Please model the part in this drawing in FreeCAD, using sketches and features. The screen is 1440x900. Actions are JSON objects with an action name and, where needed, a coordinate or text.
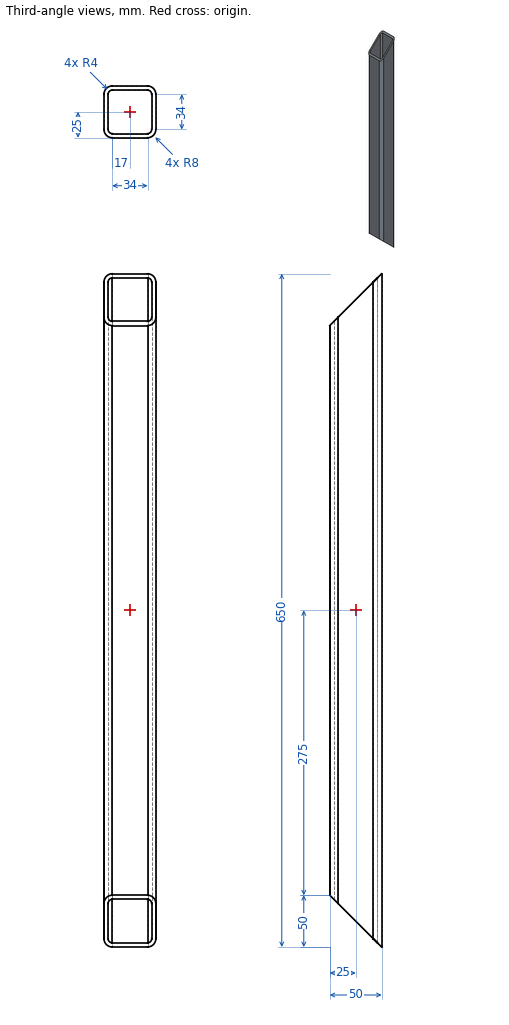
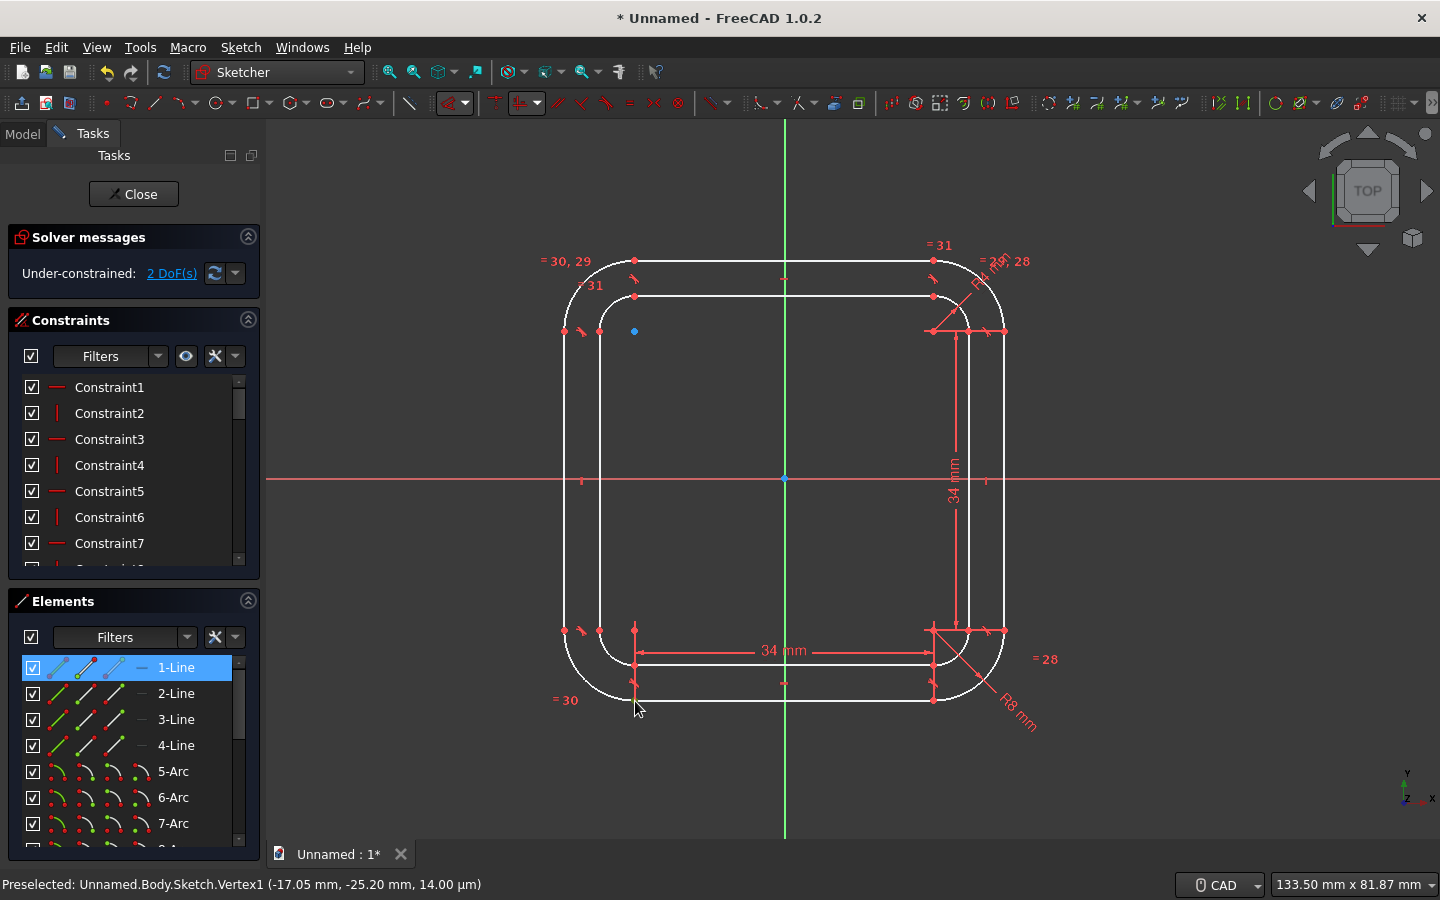
{"action": "key", "text": "l"}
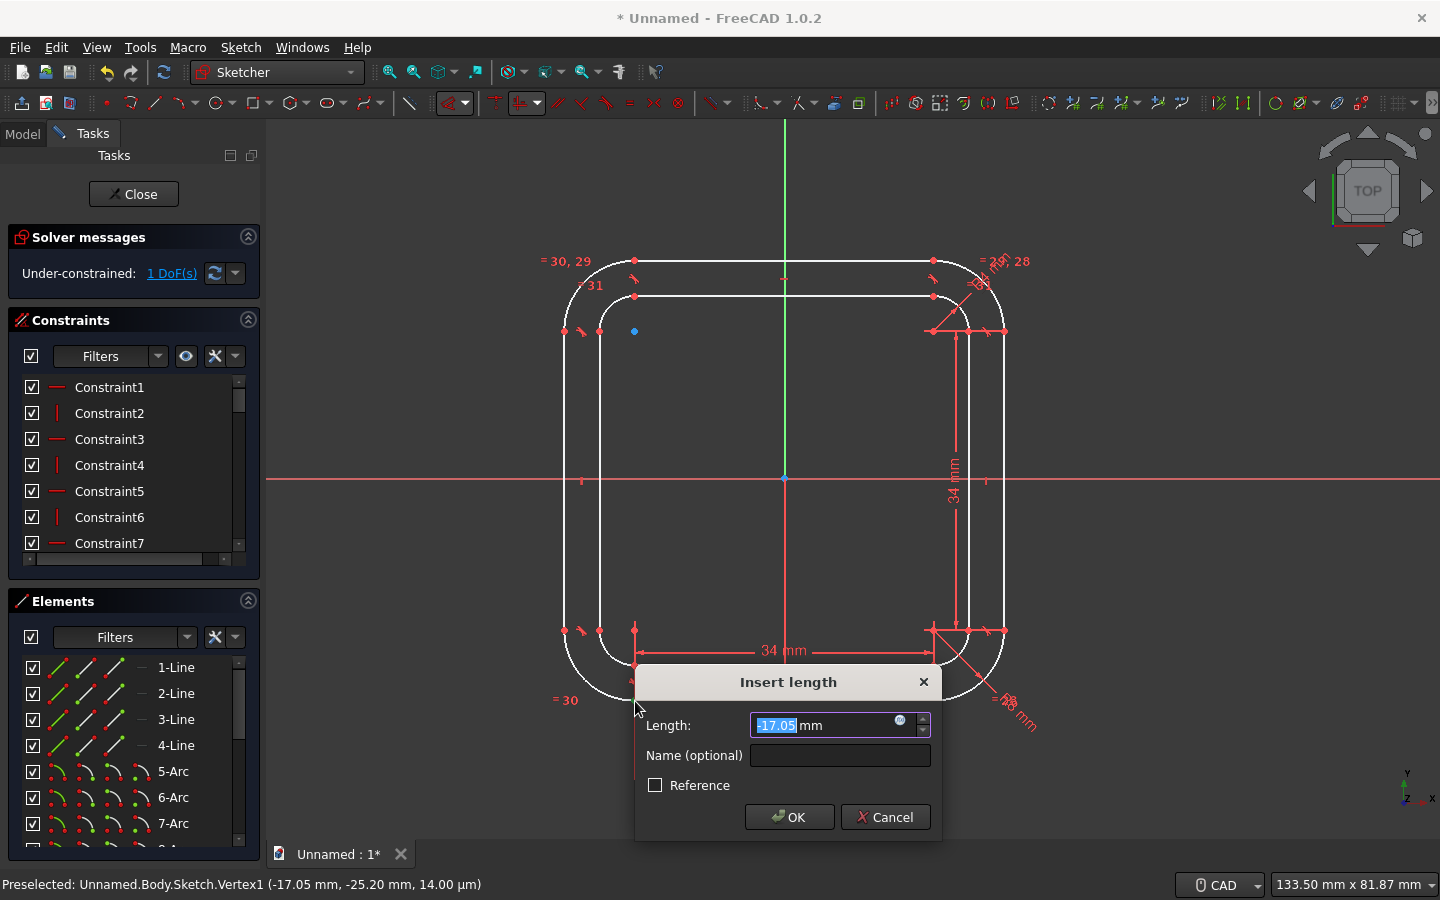
{"action": "type", "text": "-17"}
{"action": "key", "text": "Return"}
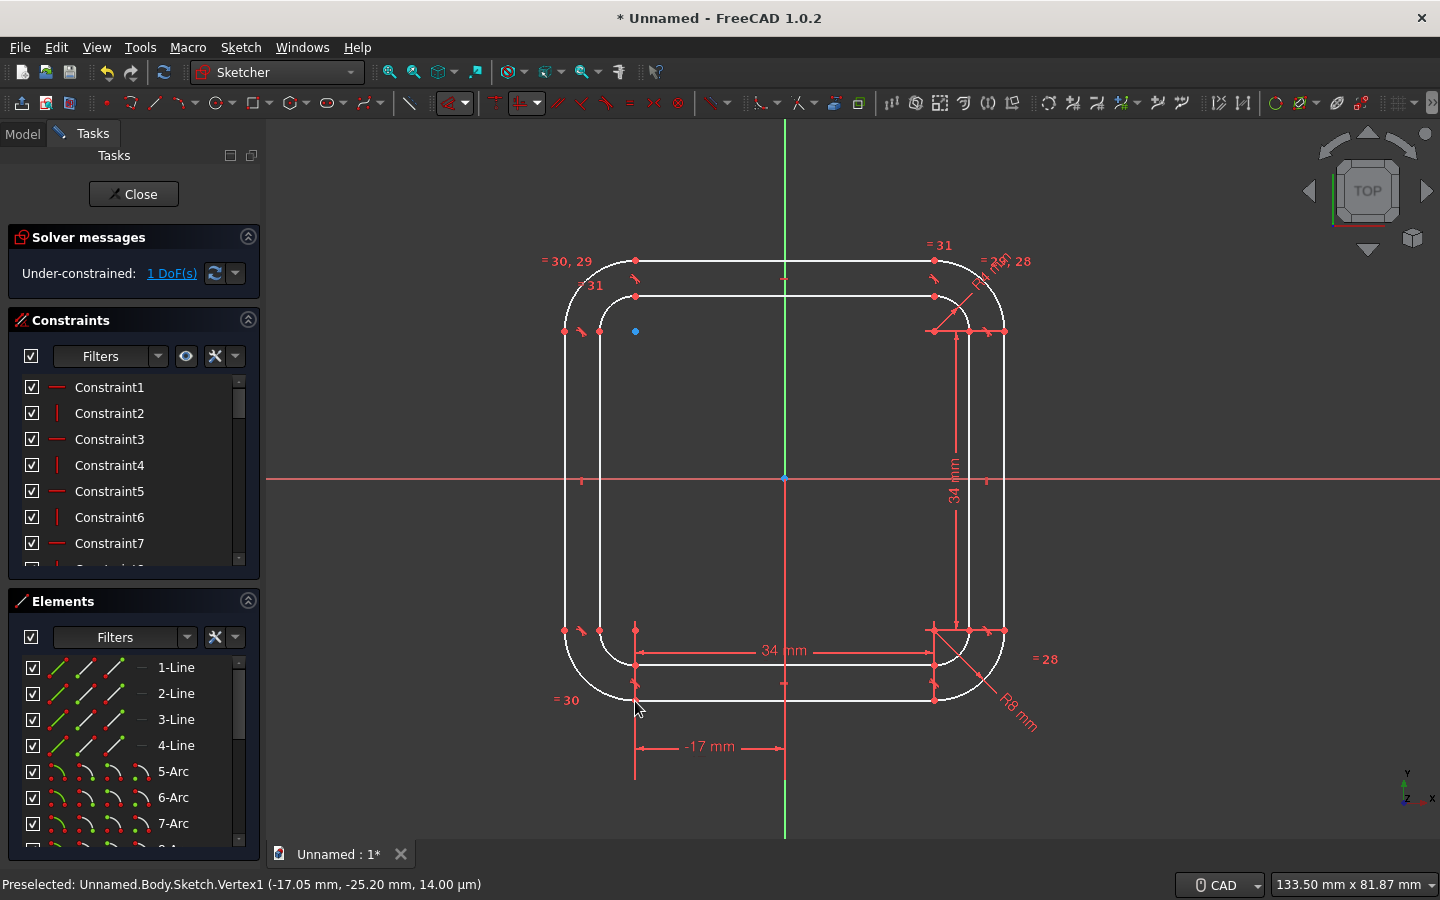
{"action": "left_click", "coordinate": [635, 701]}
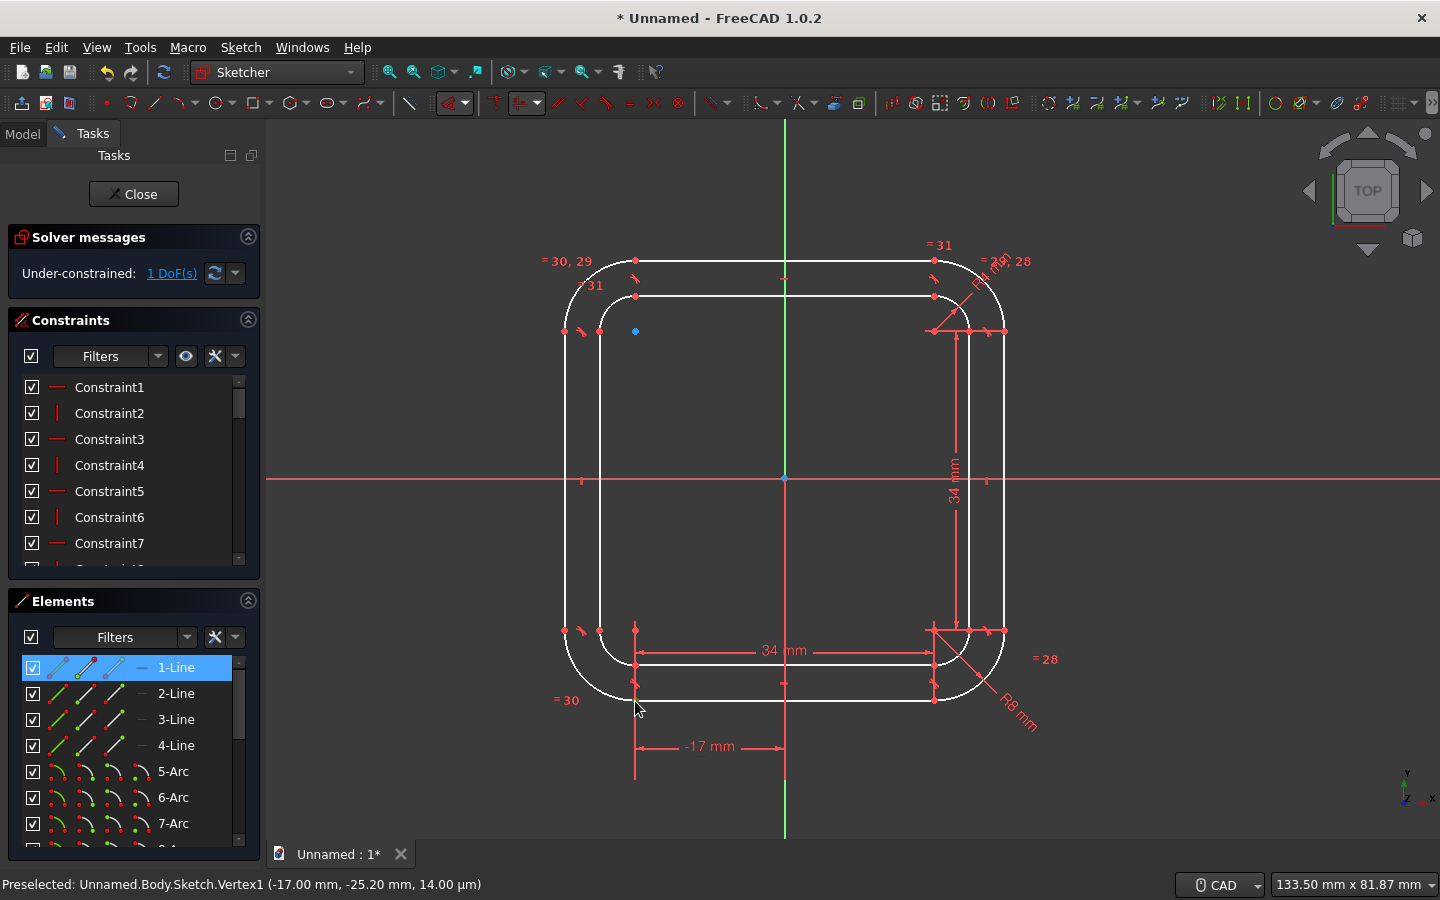
{"action": "key", "text": "i"}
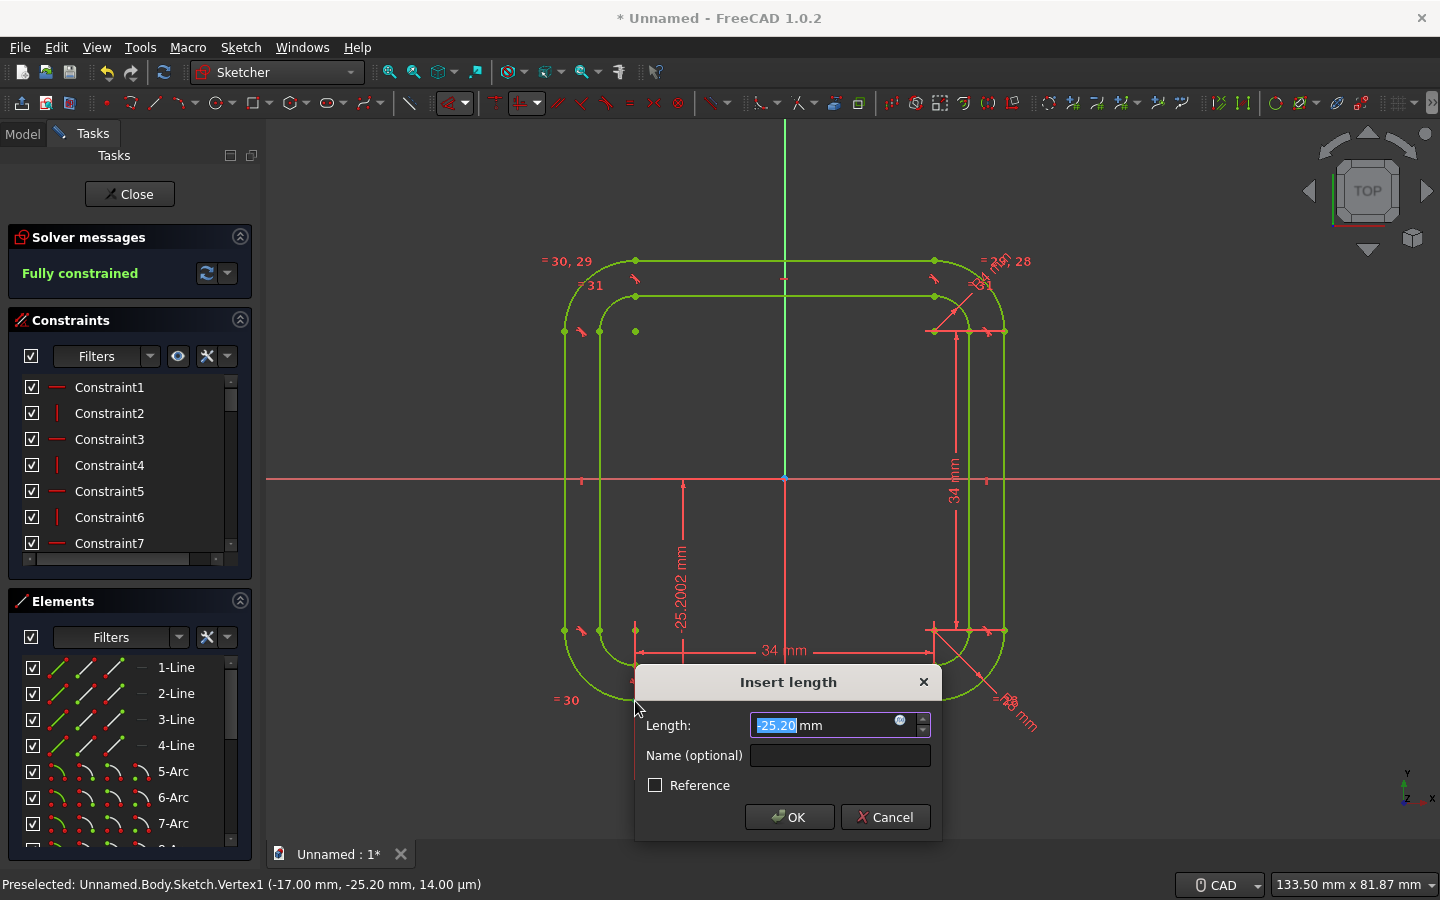
{"action": "type", "text": "-25"}
{"action": "key", "text": "Return"}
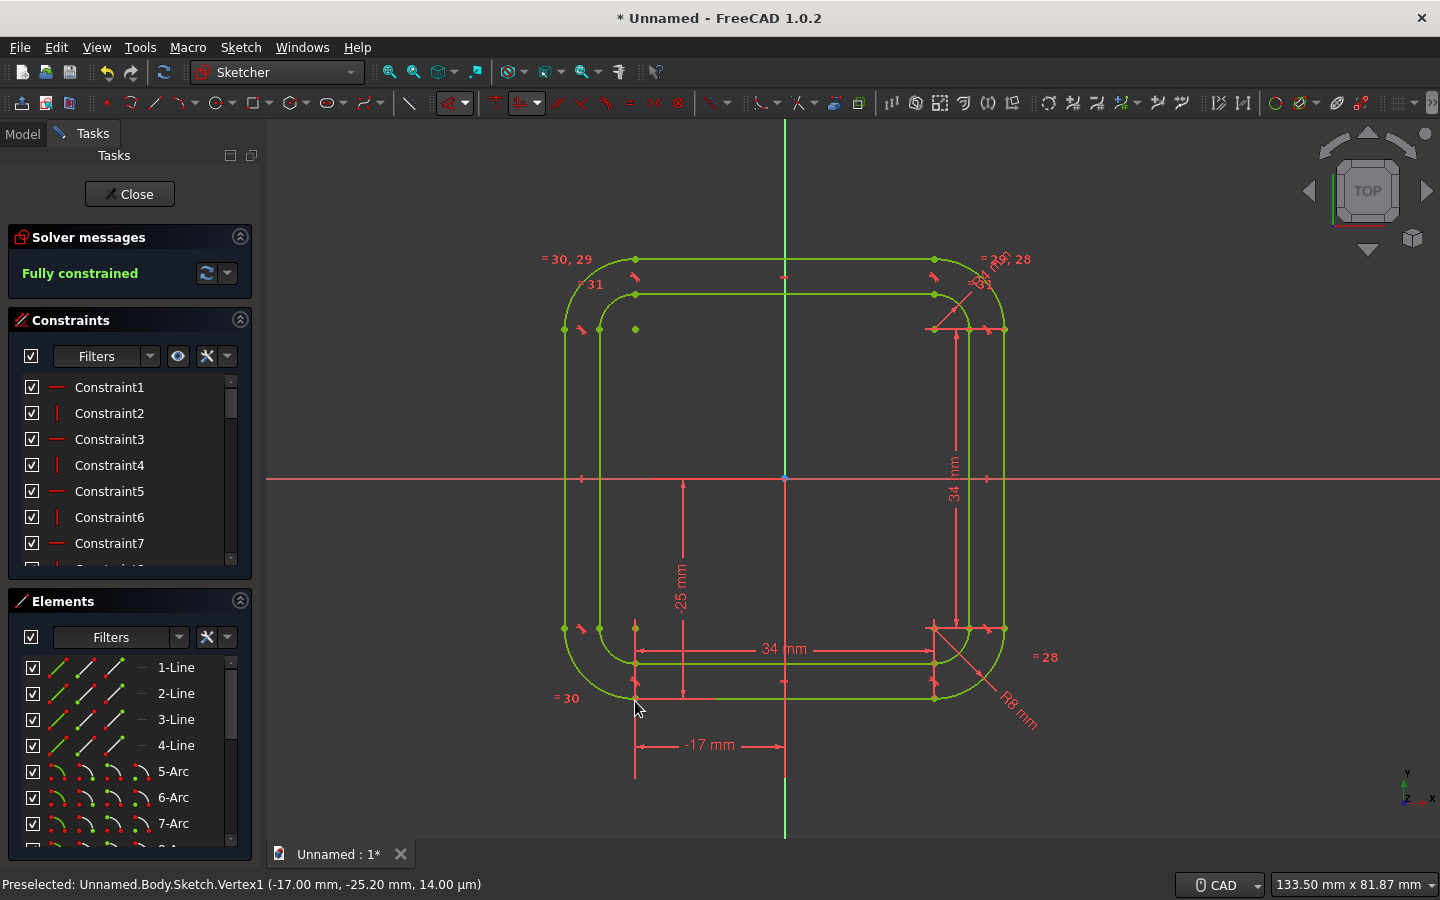
{"action": "left_click", "coordinate": [130, 194]}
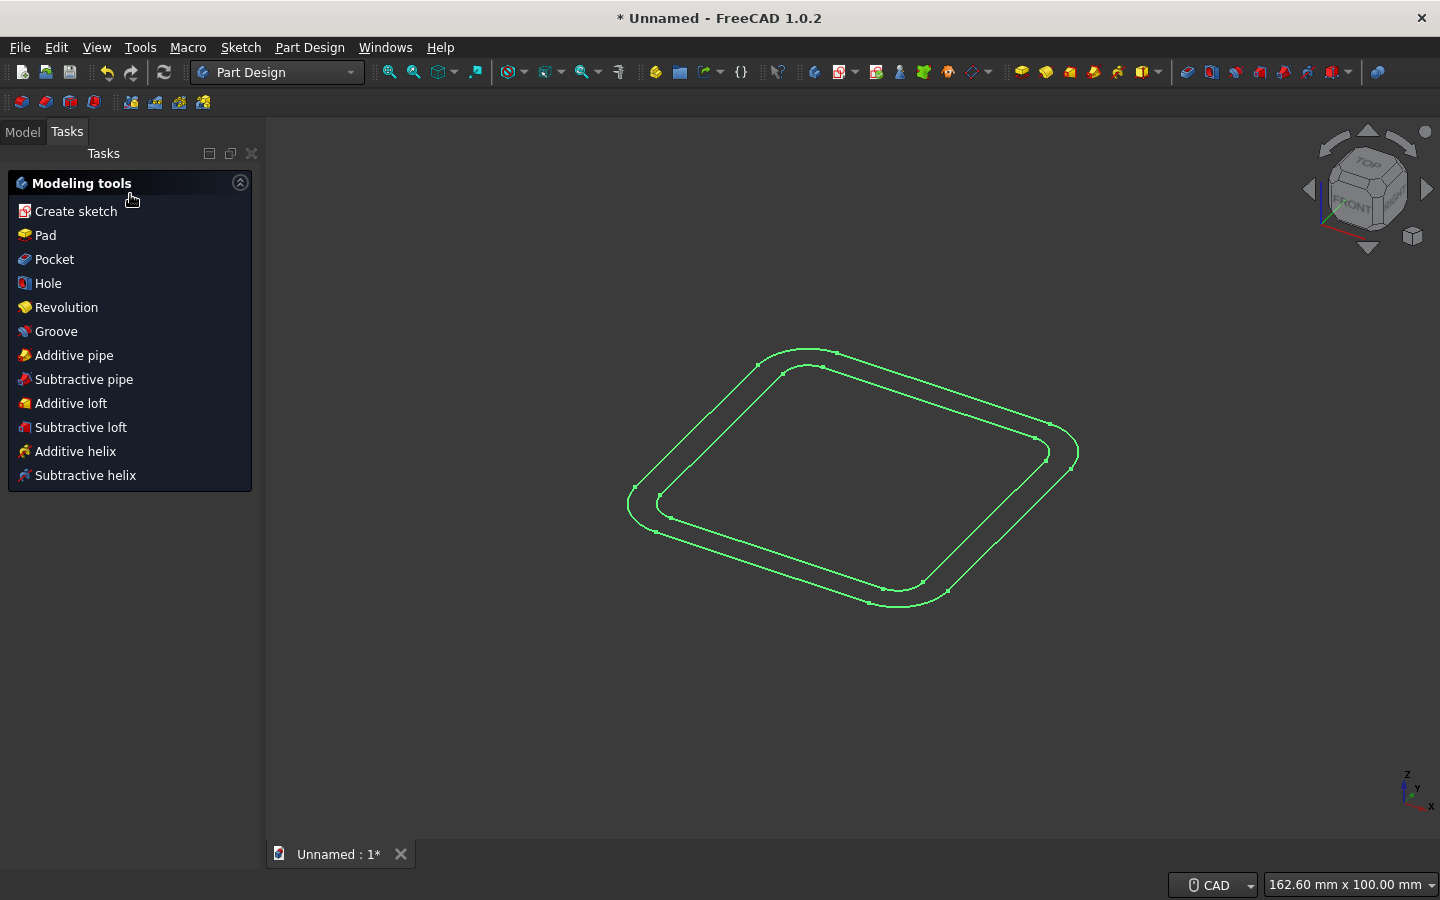
{"action": "left_click", "coordinate": [1022, 72]}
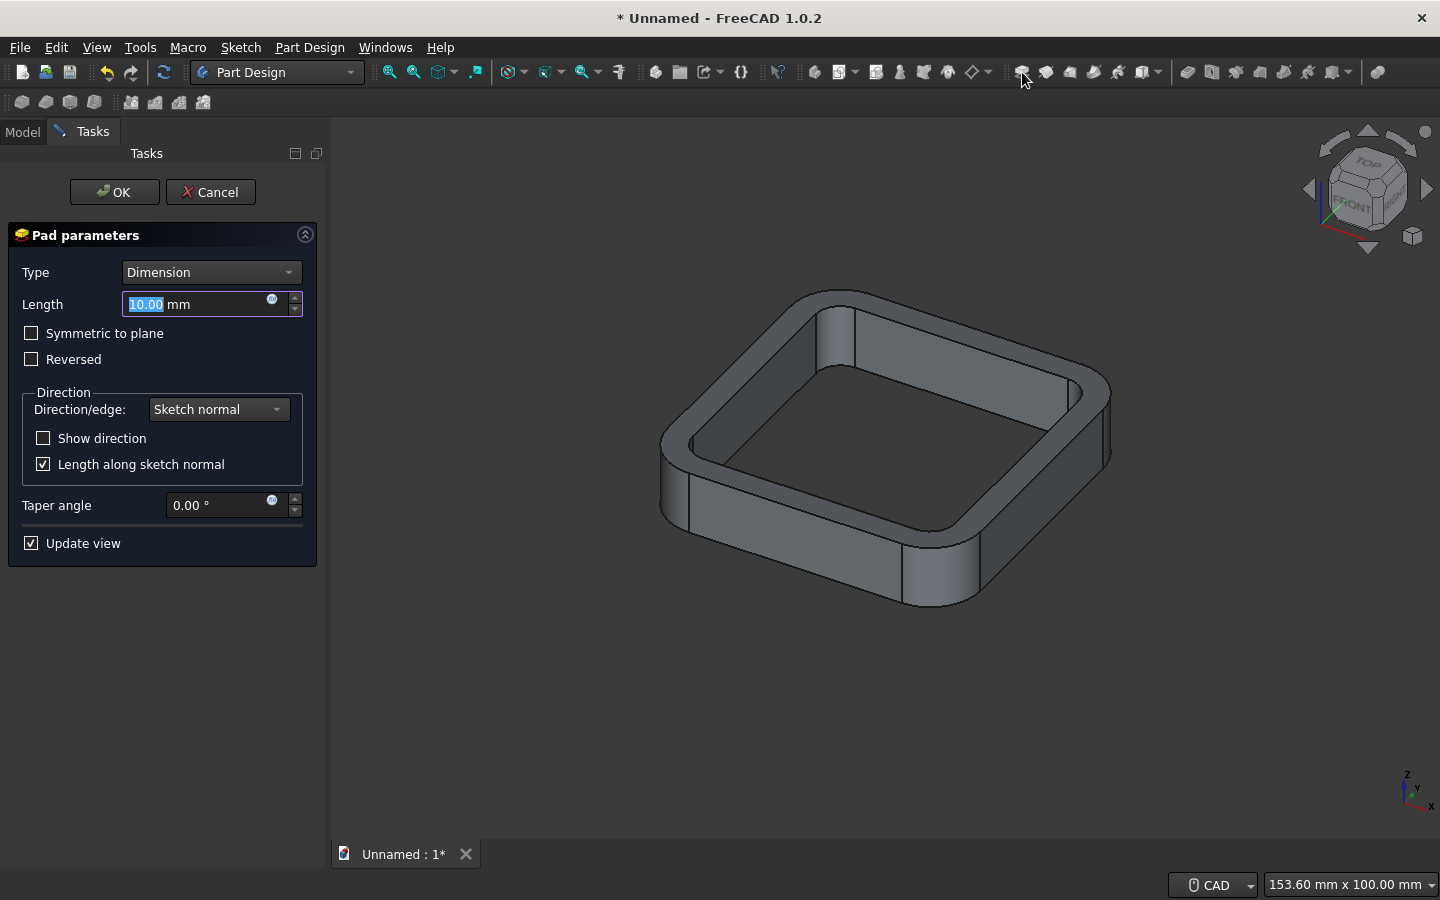
{"action": "type", "text": "650"}
{"action": "key", "text": "Tab"}